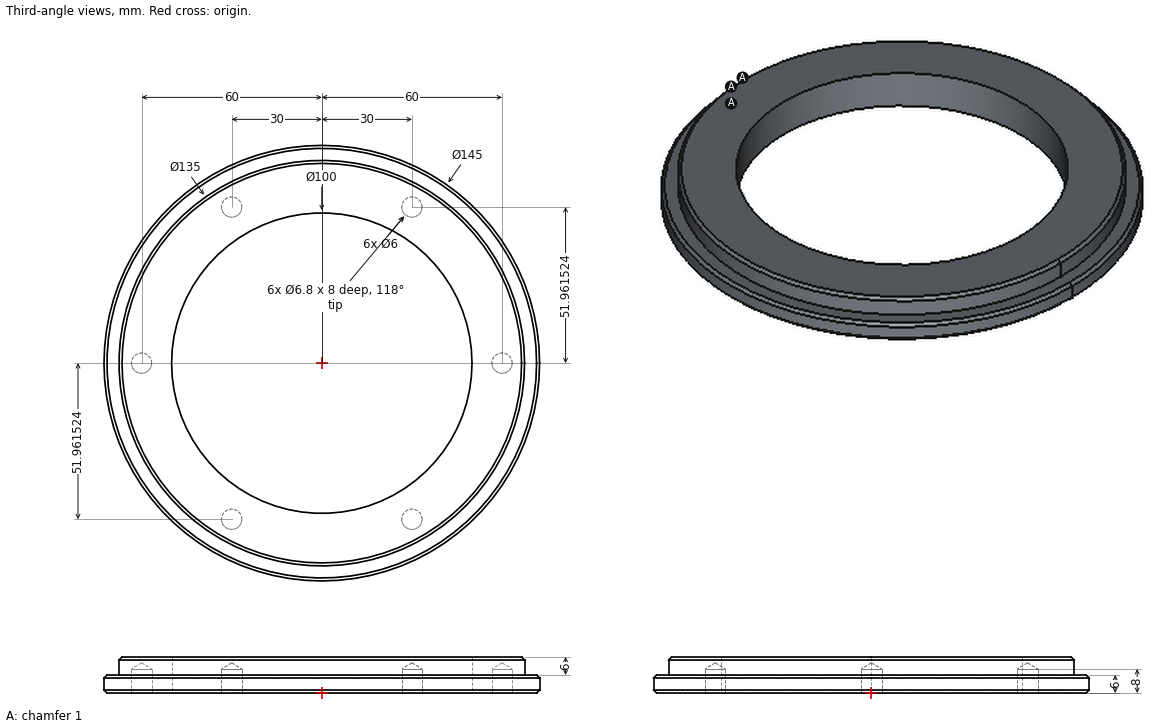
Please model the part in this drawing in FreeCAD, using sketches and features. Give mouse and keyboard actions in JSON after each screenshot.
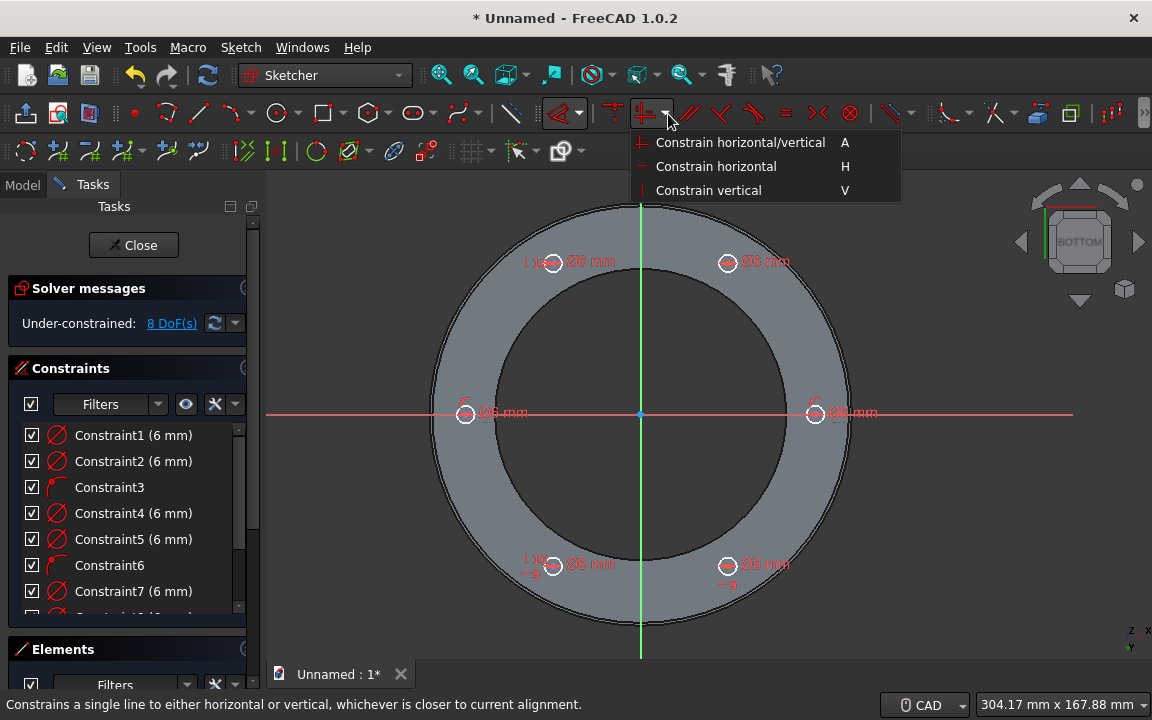
{"action": "left_click", "coordinate": [766, 190]}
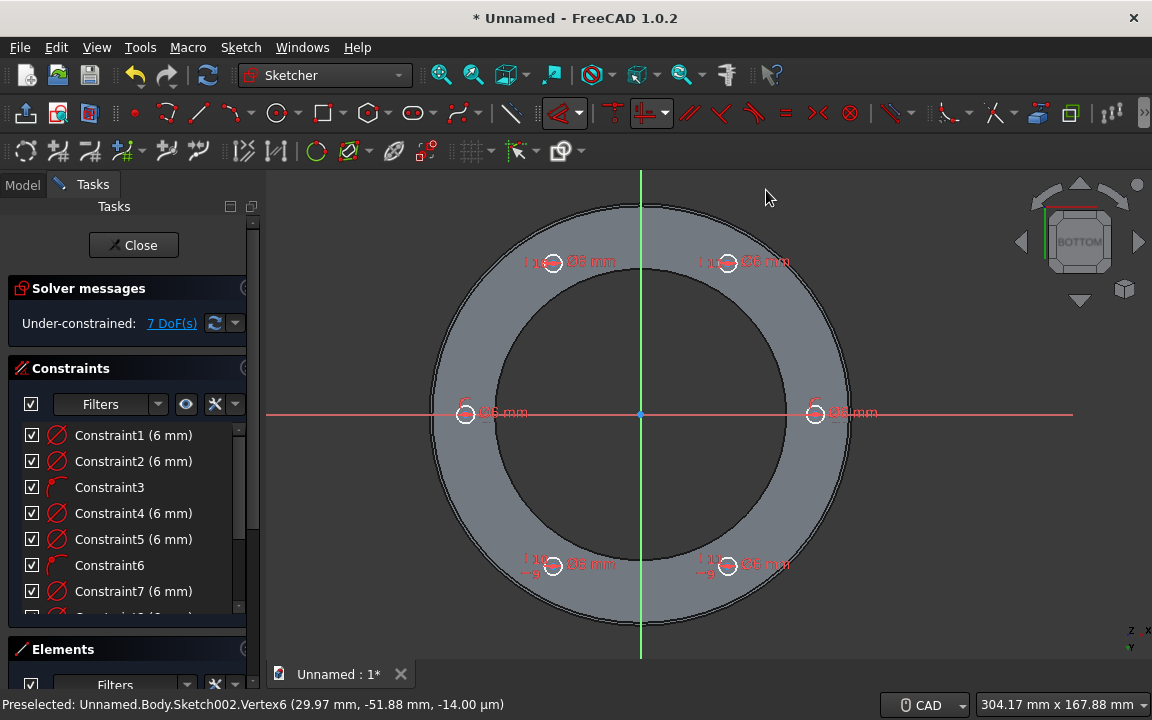
{"action": "left_click", "coordinate": [553, 263]}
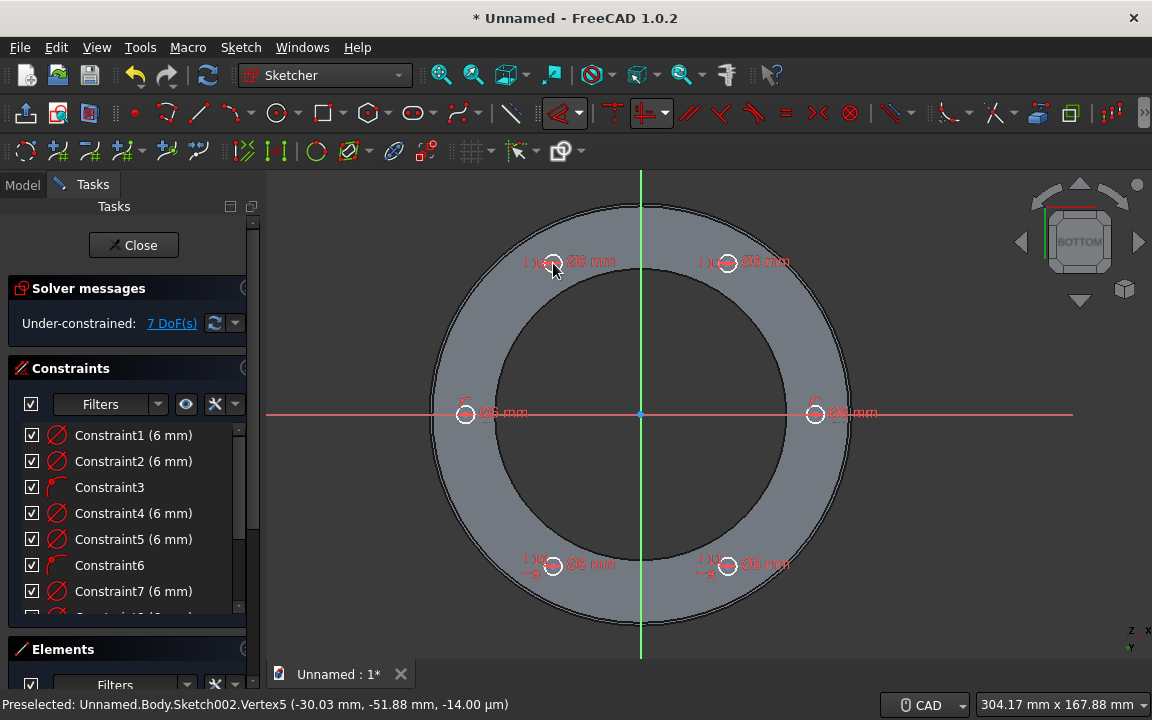
{"action": "left_click", "coordinate": [728, 263]}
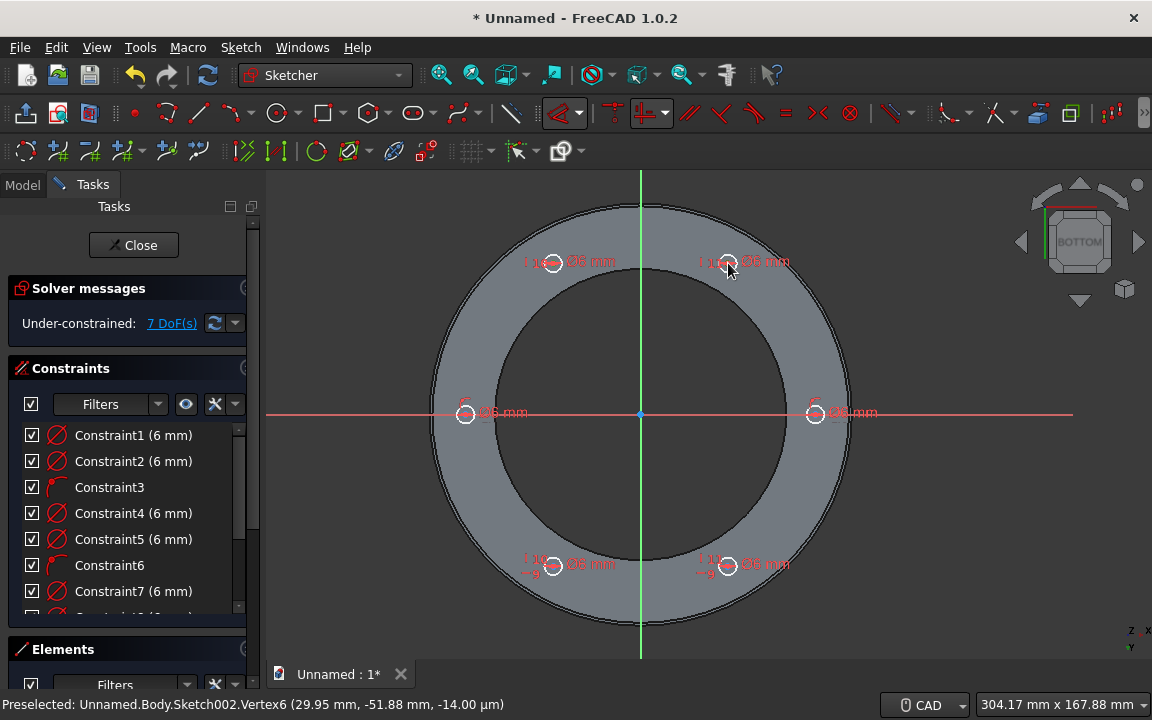
{"action": "key", "text": "h"}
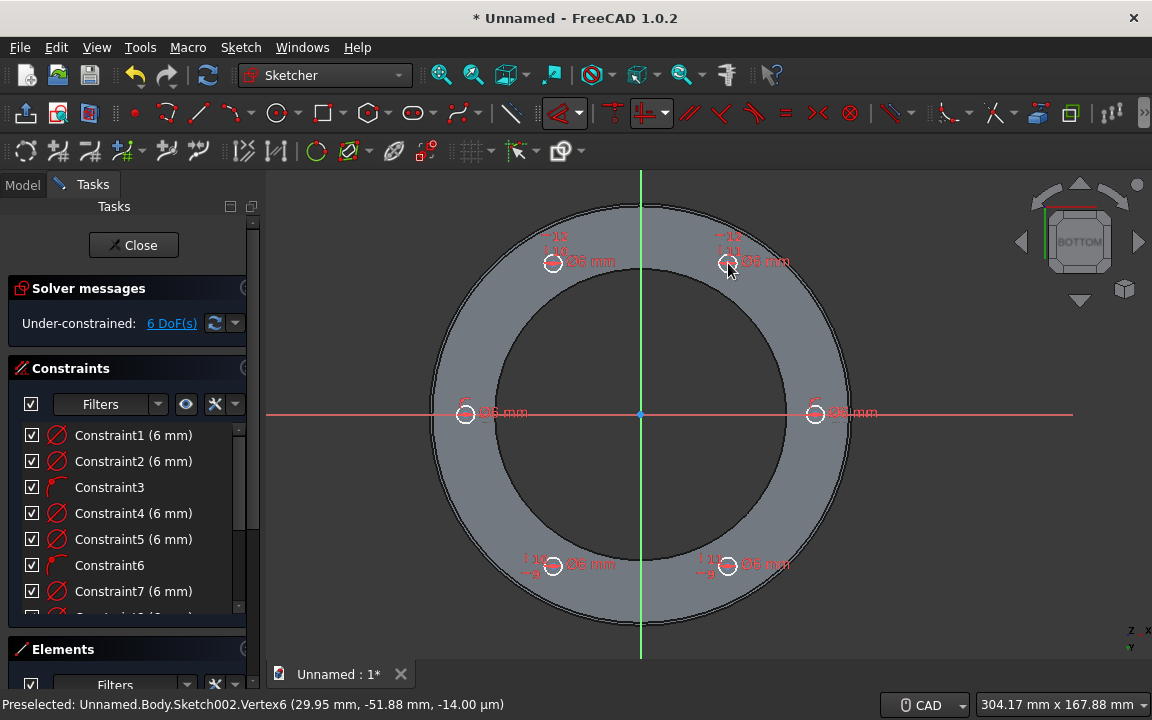
{"action": "left_click", "coordinate": [728, 566]}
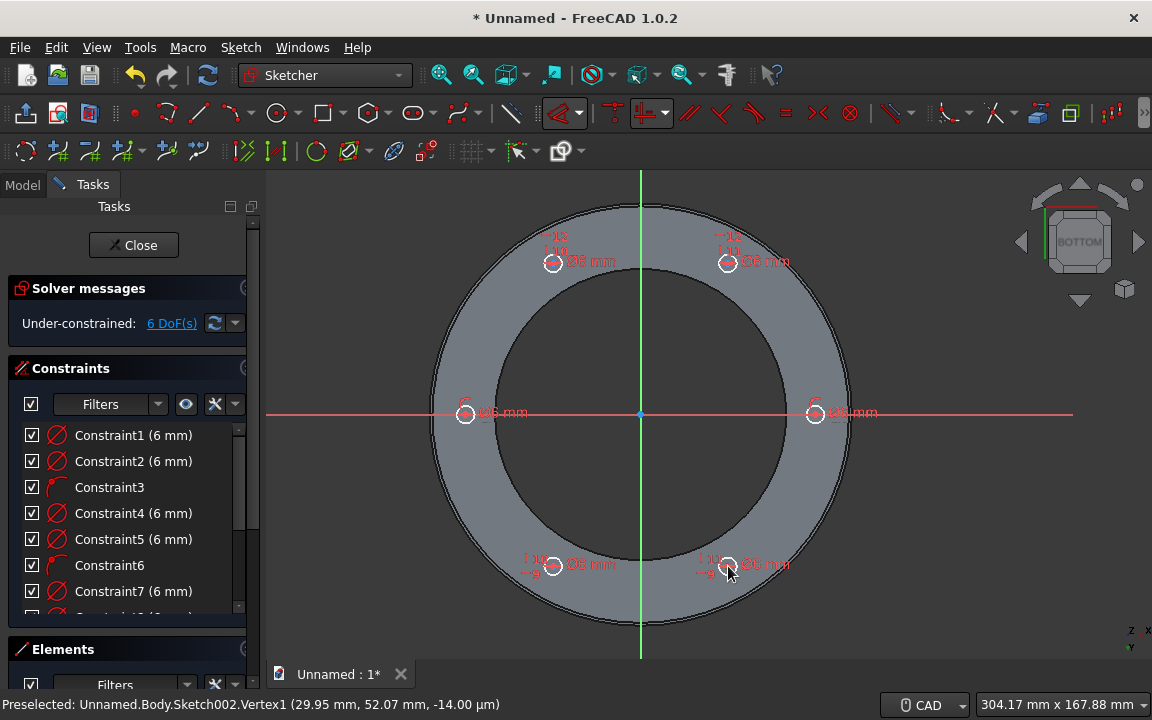
{"action": "left_click", "coordinate": [582, 114]}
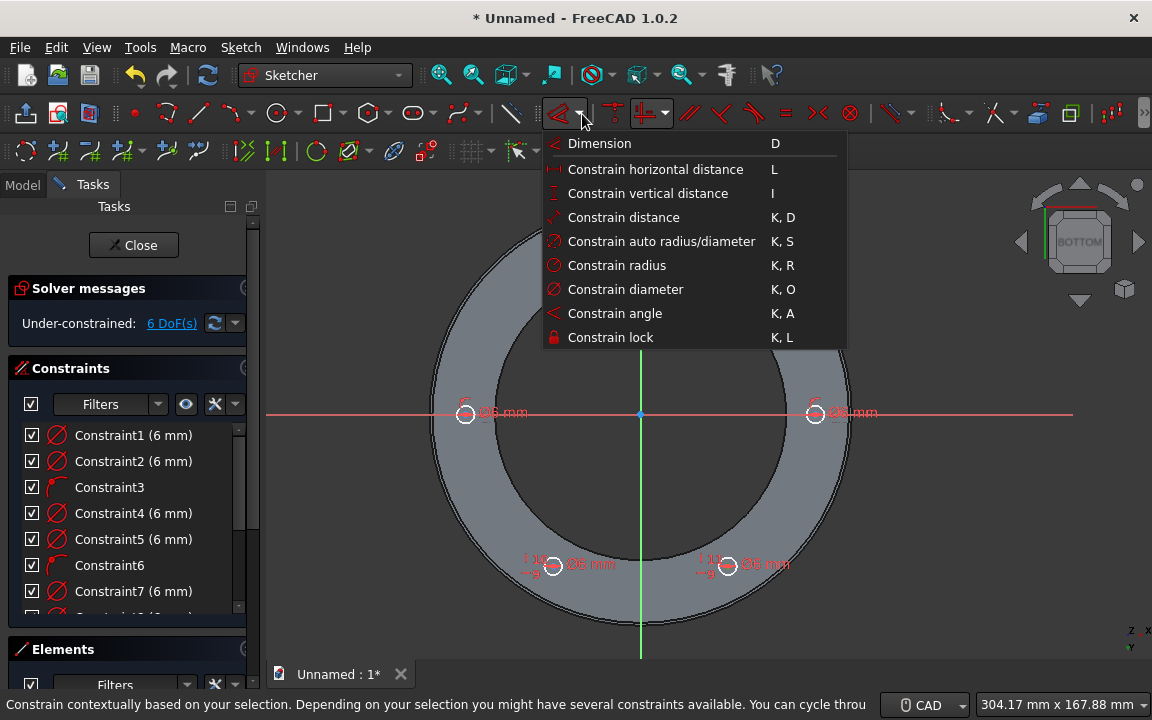
{"action": "left_click", "coordinate": [695, 169]}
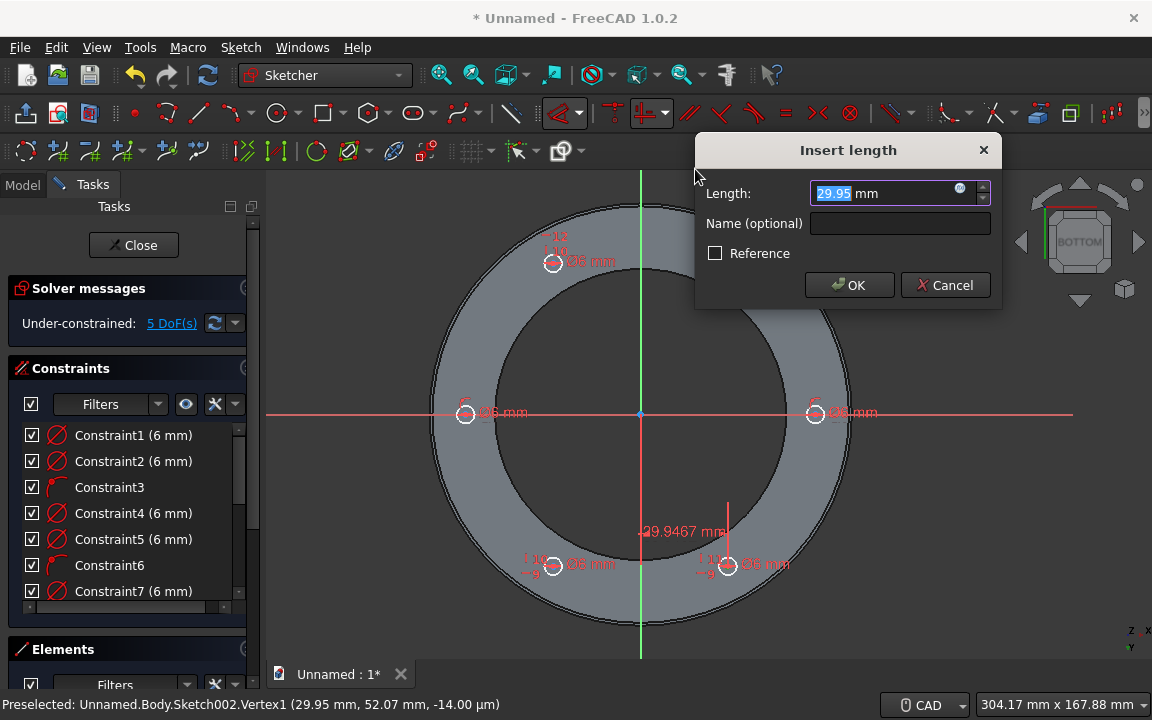
{"action": "type", "text": "30"}
{"action": "key", "text": "Return"}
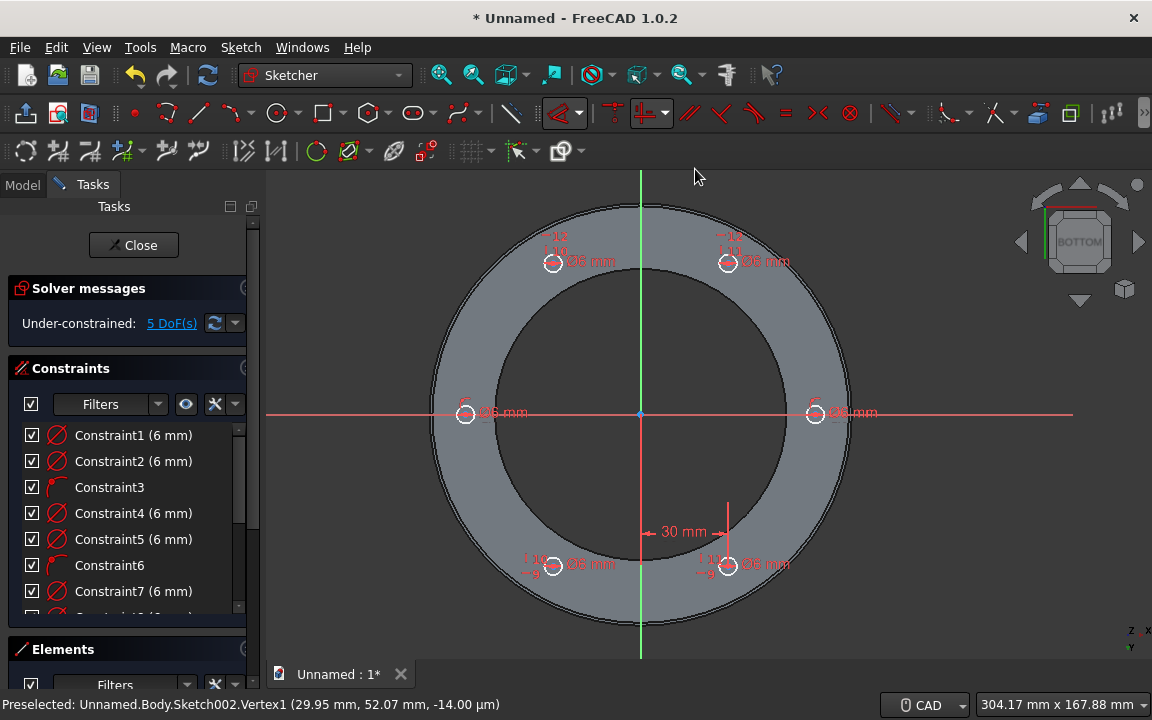
{"action": "left_click", "coordinate": [815, 415]}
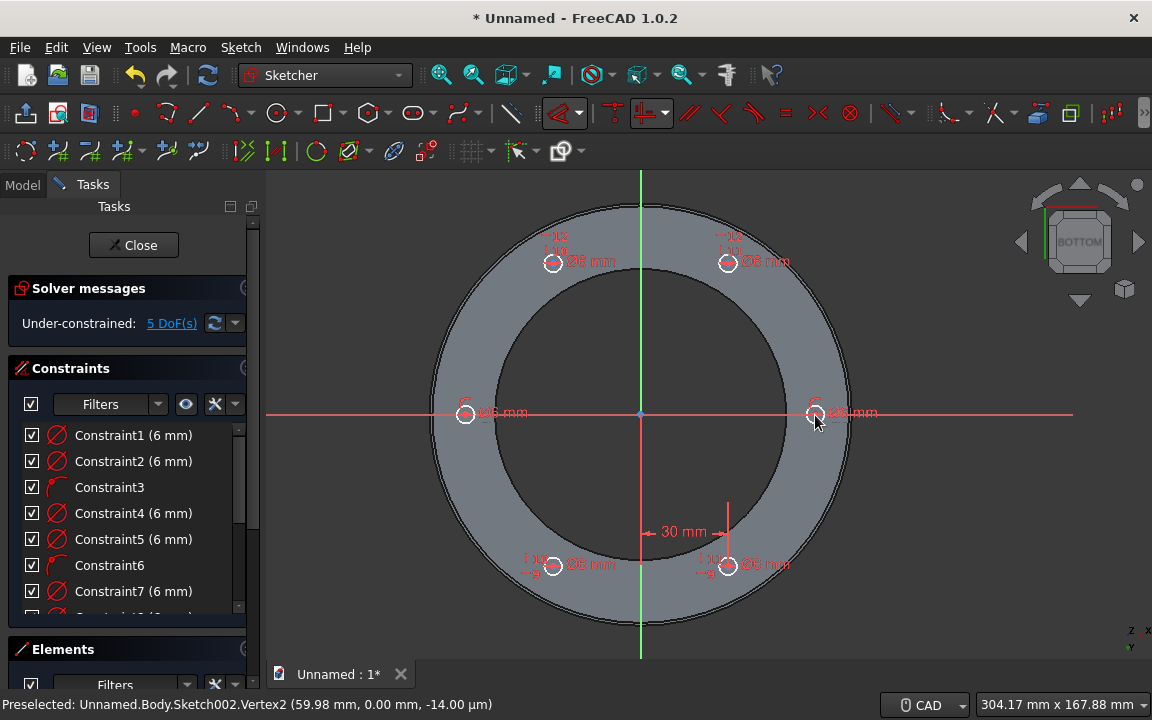
{"action": "left_click", "coordinate": [582, 114]}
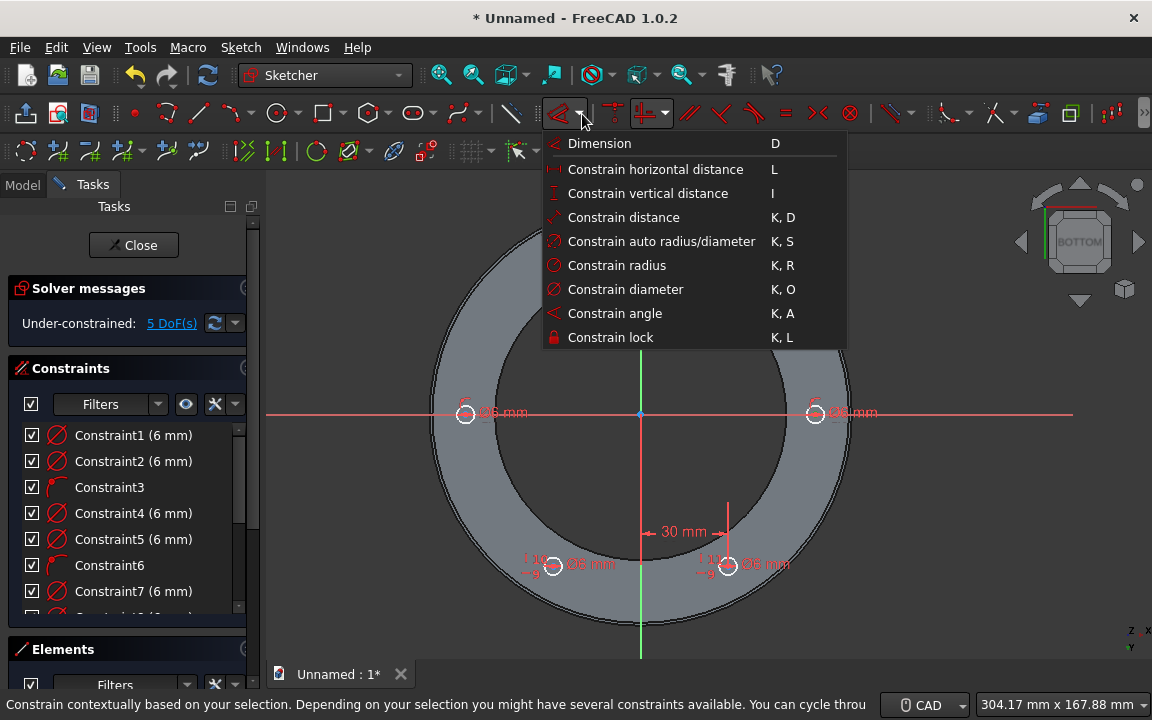
{"action": "left_click", "coordinate": [695, 169]}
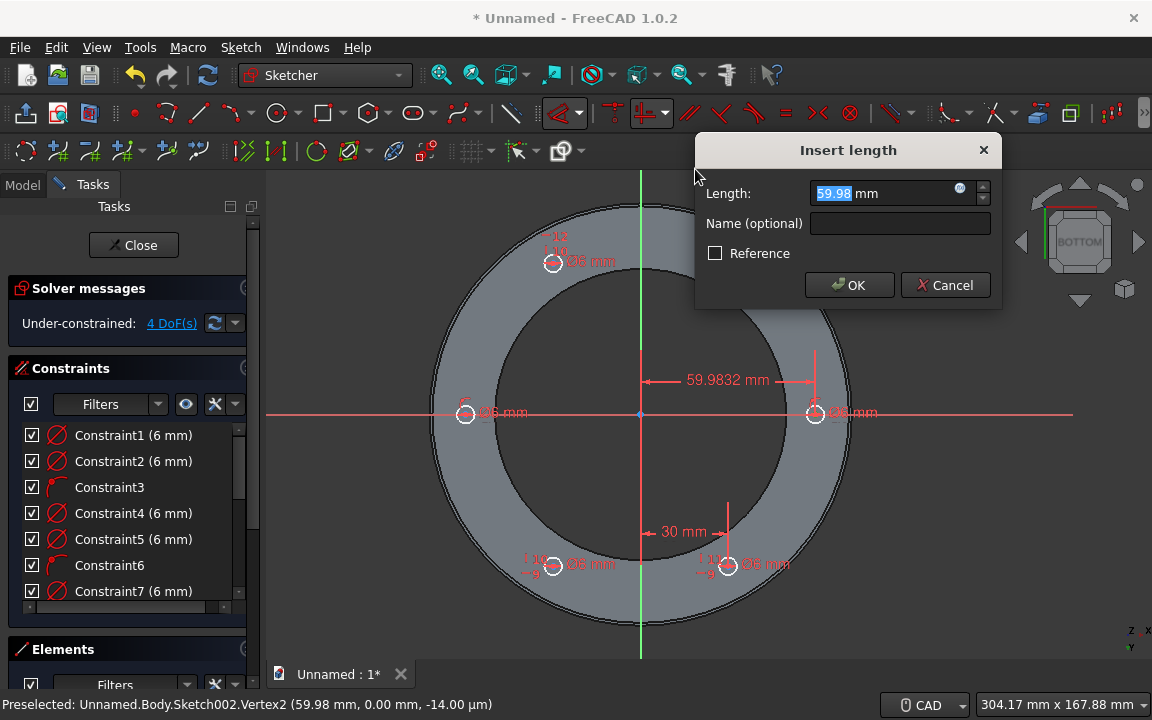
{"action": "type", "text": "60"}
{"action": "key", "text": "Return"}